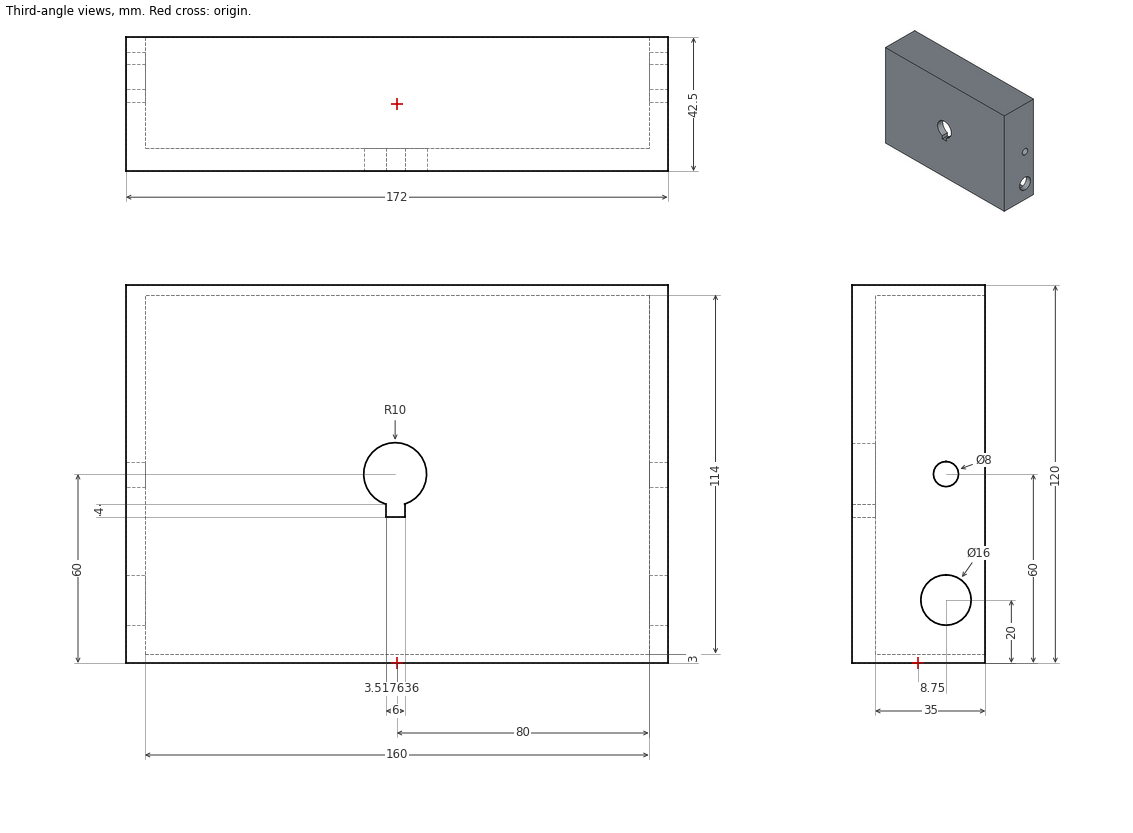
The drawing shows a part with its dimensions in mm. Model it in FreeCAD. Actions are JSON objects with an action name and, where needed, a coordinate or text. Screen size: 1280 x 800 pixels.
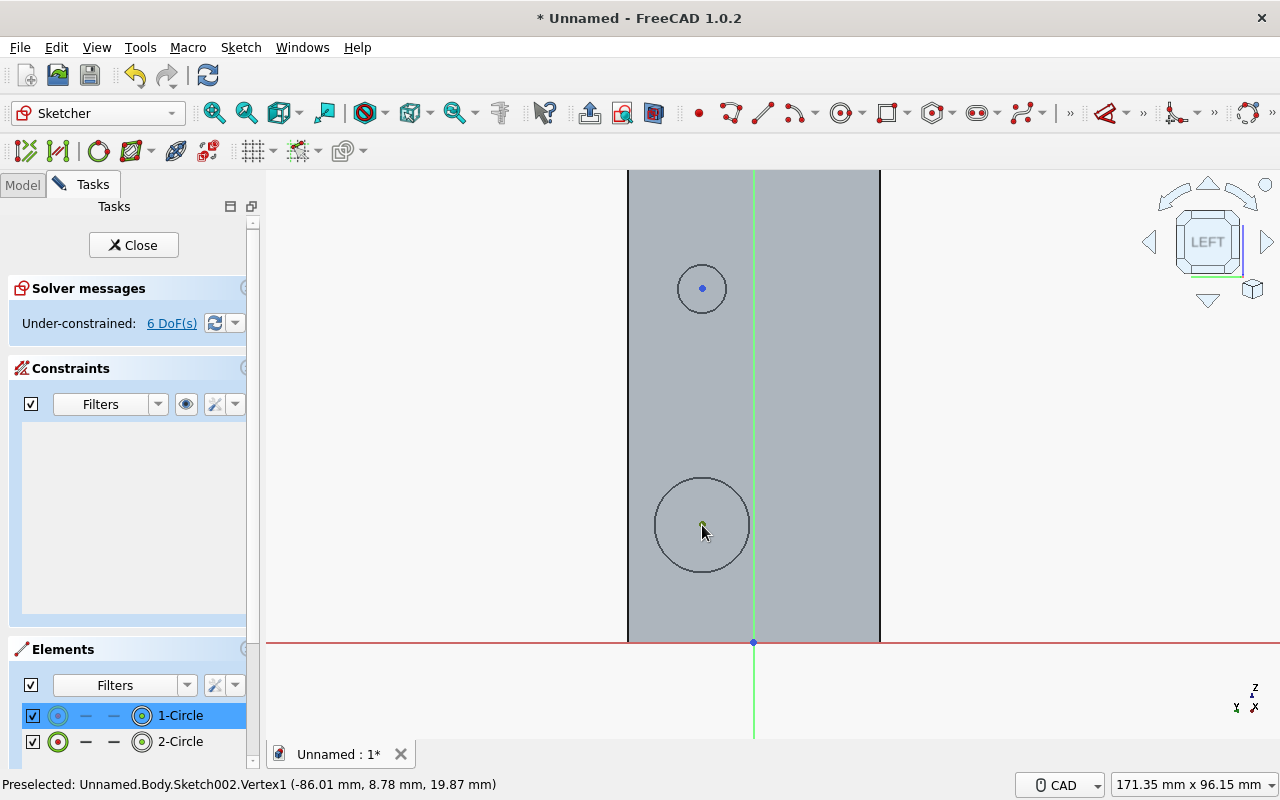
{"action": "left_click", "coordinate": [702, 289]}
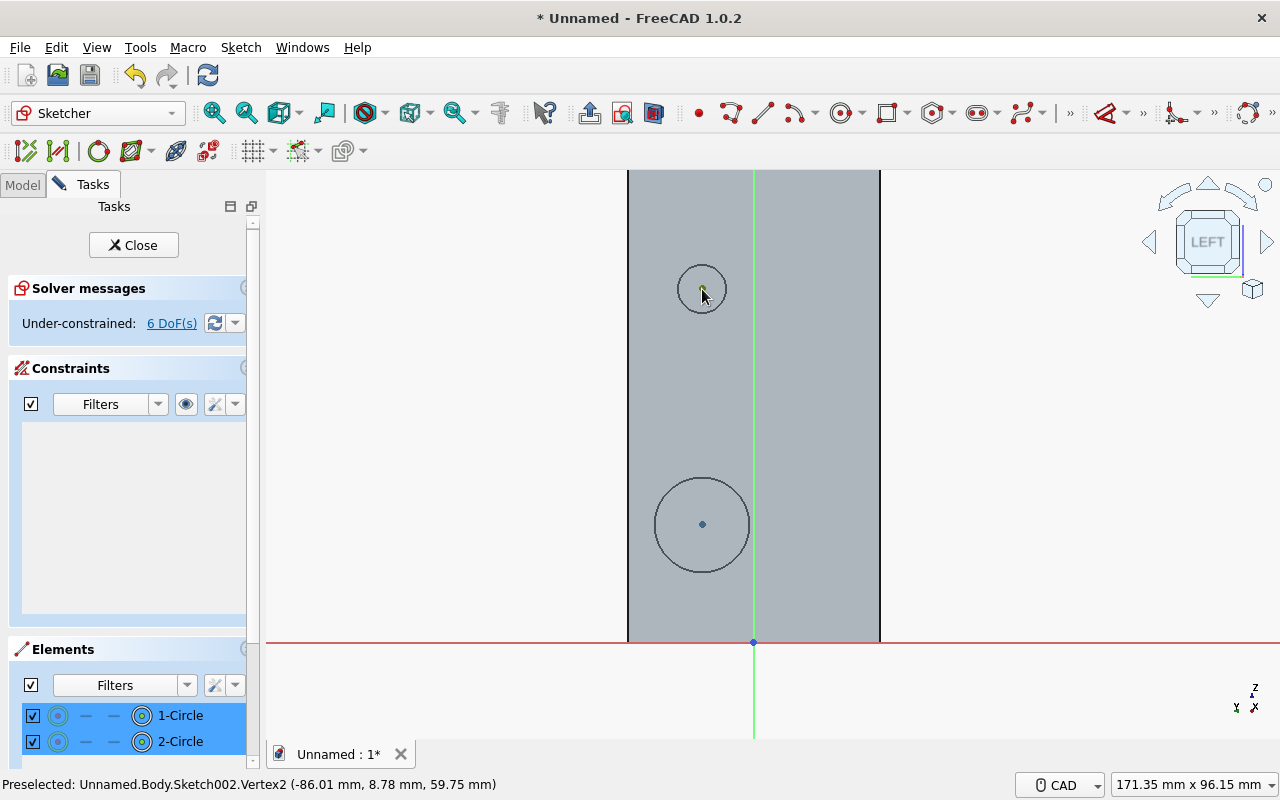
{"action": "key", "text": "v"}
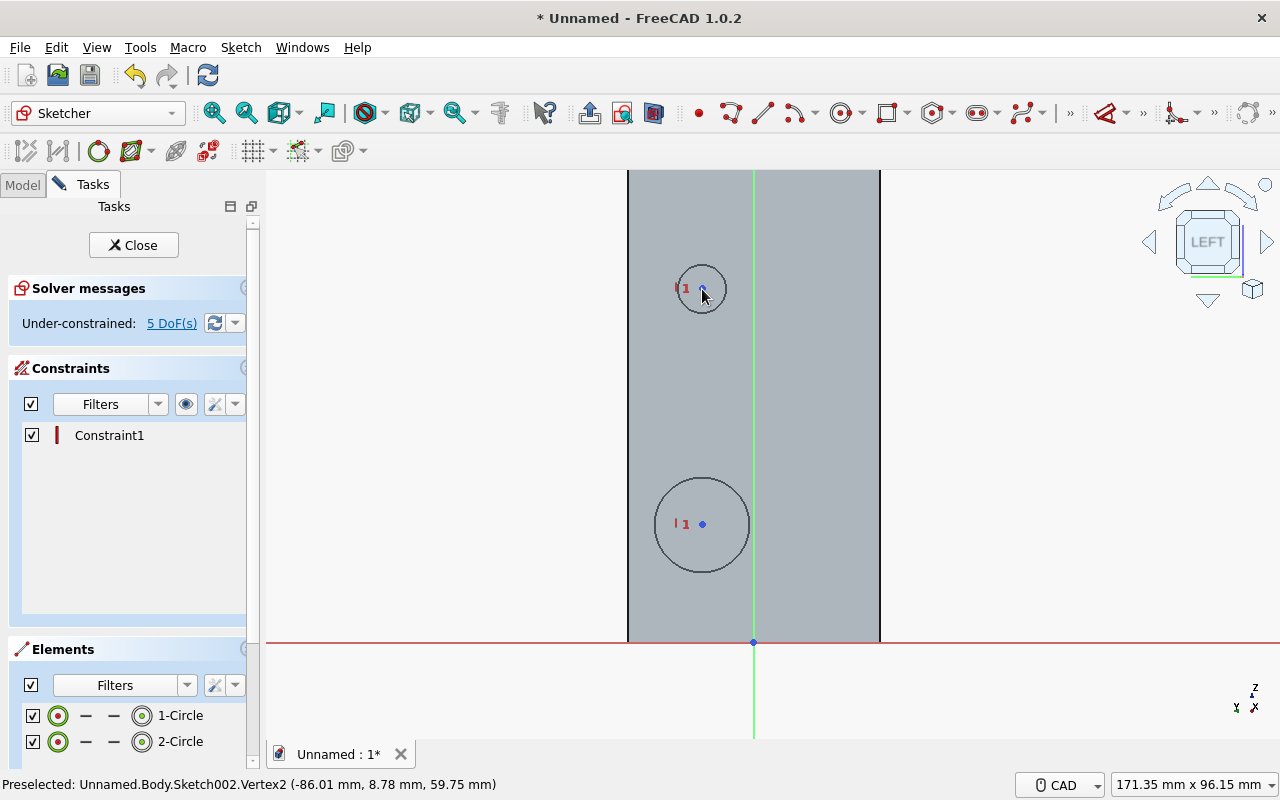
{"action": "left_click", "coordinate": [1106, 114]}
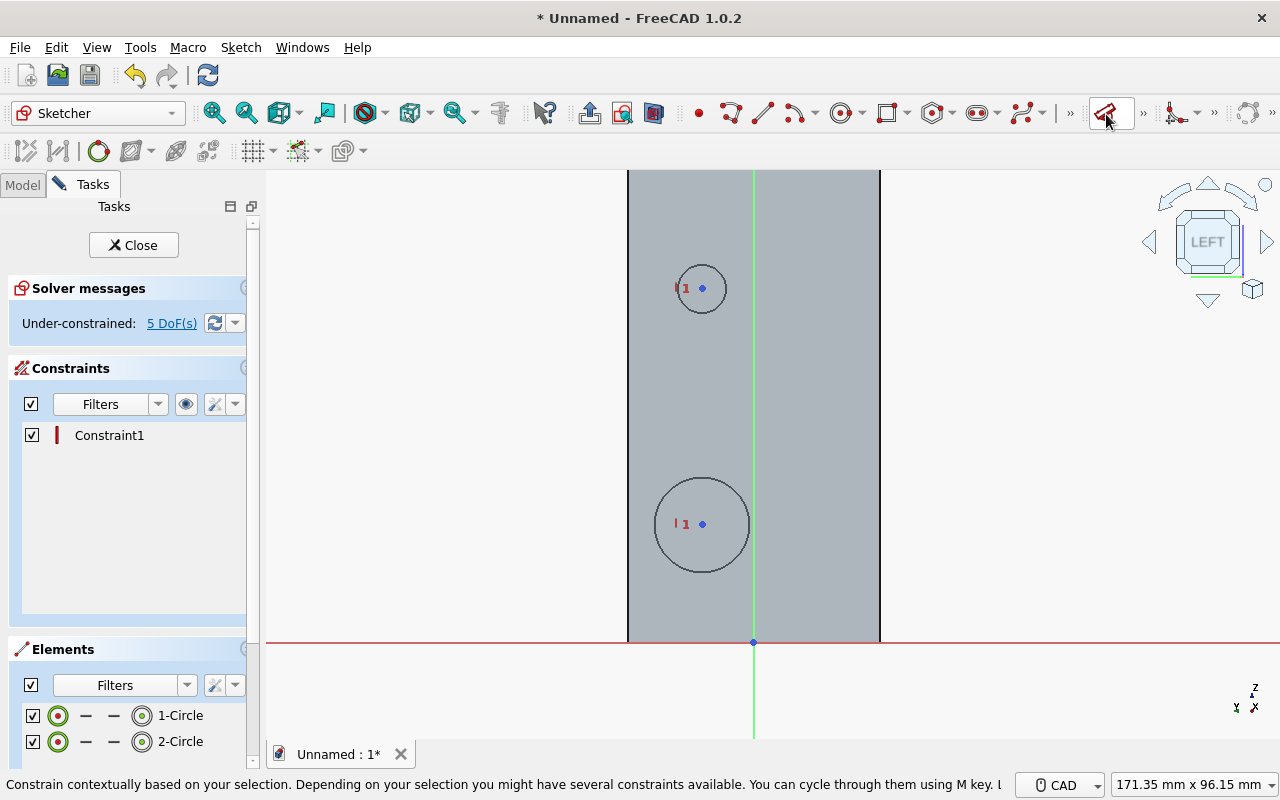
{"action": "left_click", "coordinate": [735, 491]}
{"action": "left_click", "coordinate": [778, 502]}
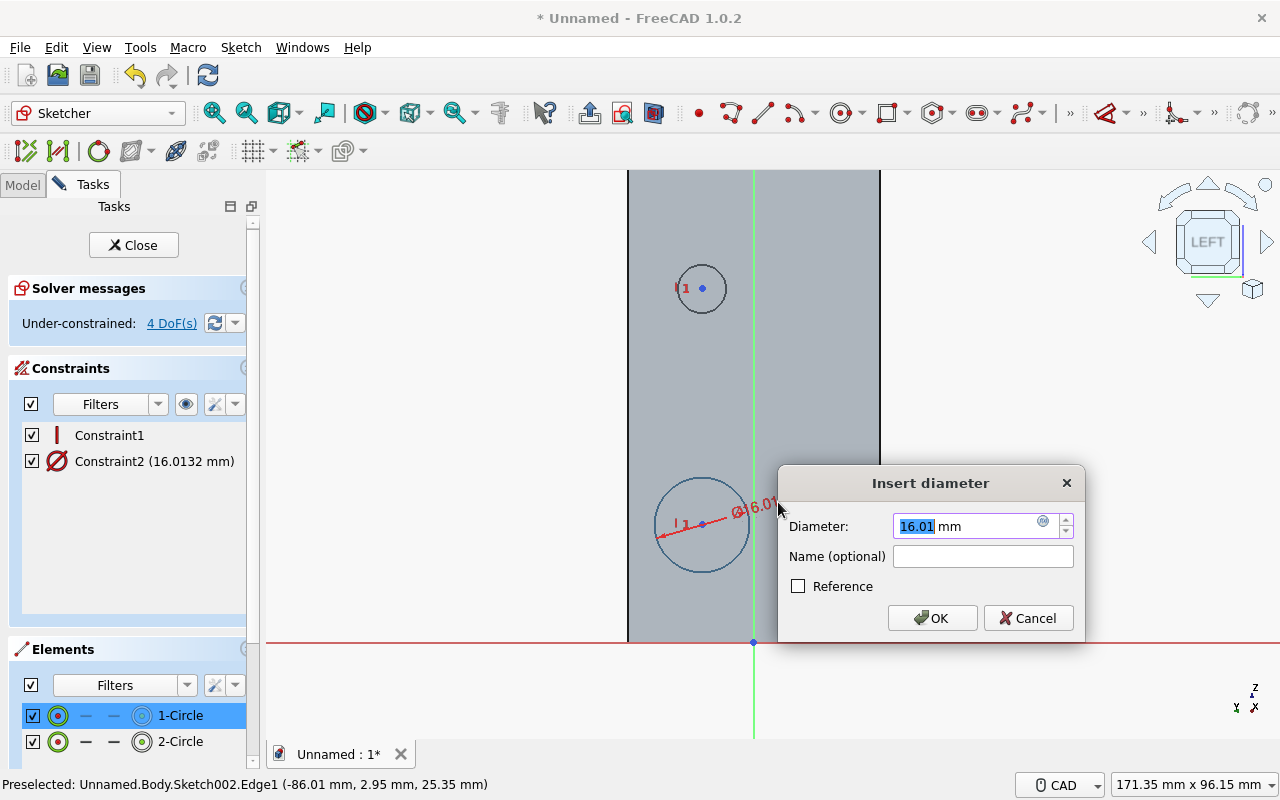
{"action": "type", "text": "16"}
{"action": "key", "text": "Return"}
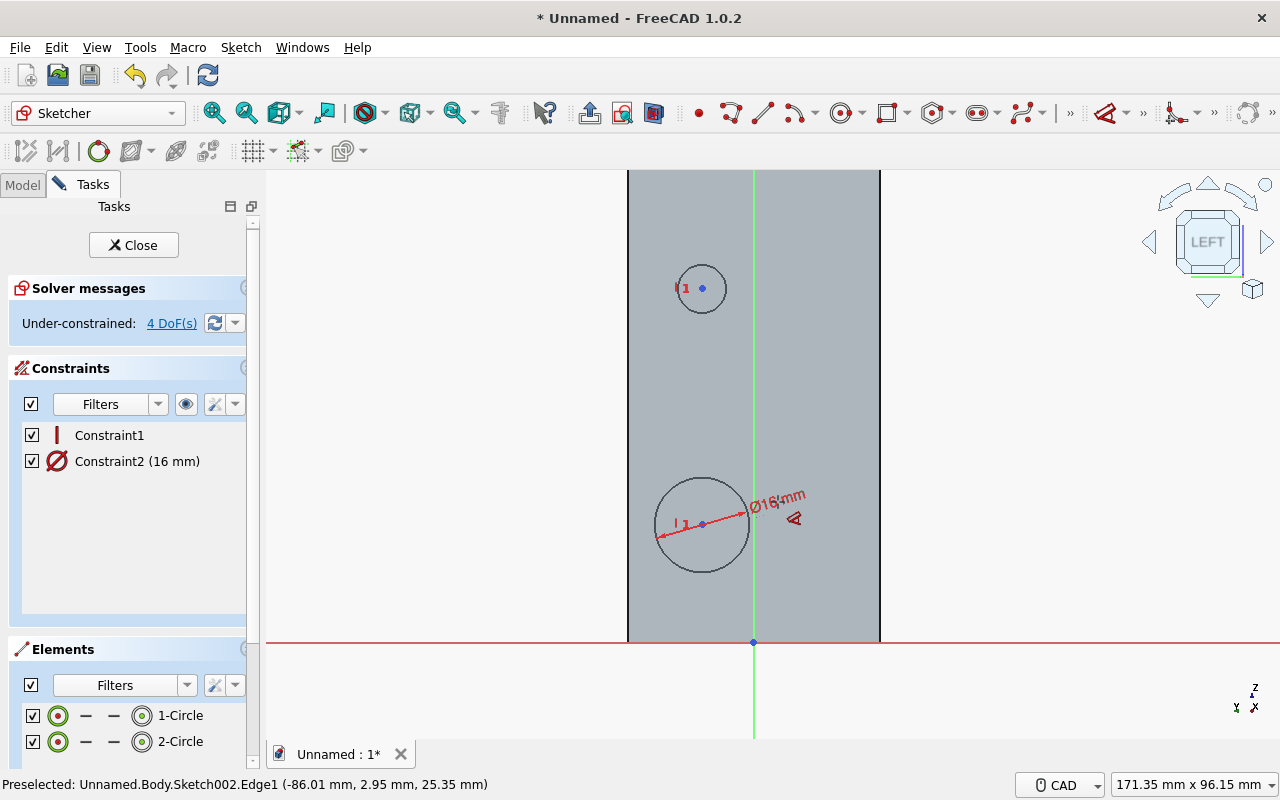
{"action": "left_click", "coordinate": [719, 272]}
{"action": "left_click", "coordinate": [718, 235]}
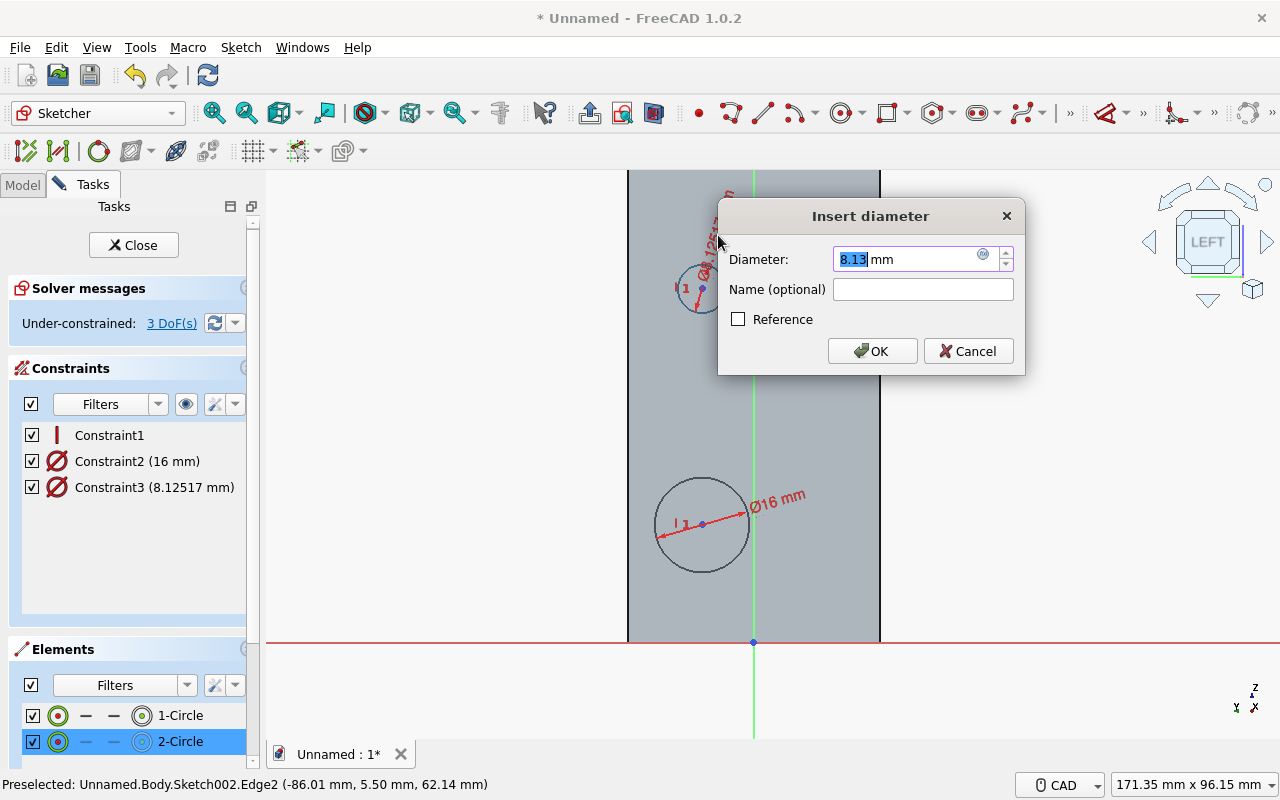
{"action": "type", "text": "8"}
{"action": "key", "text": "Return"}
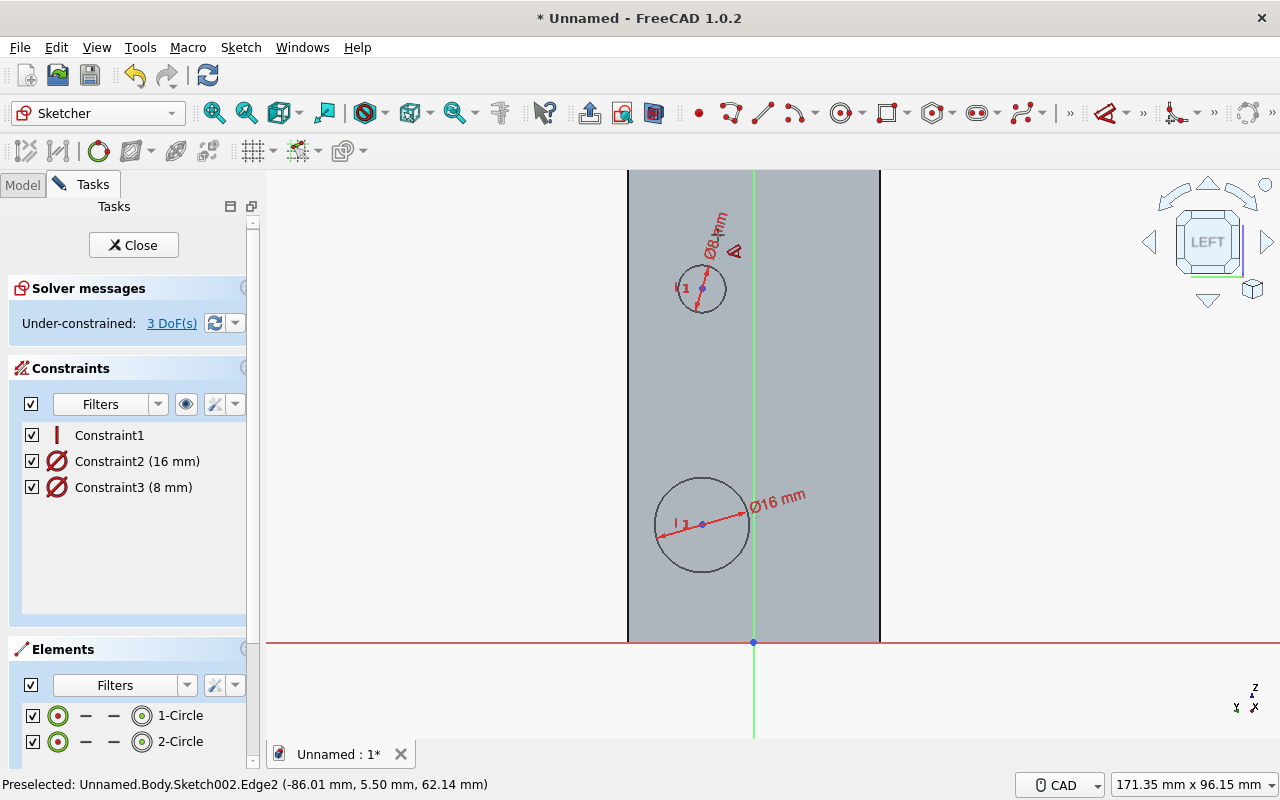
{"action": "left_click", "coordinate": [702, 525]}
{"action": "left_click", "coordinate": [788, 584]}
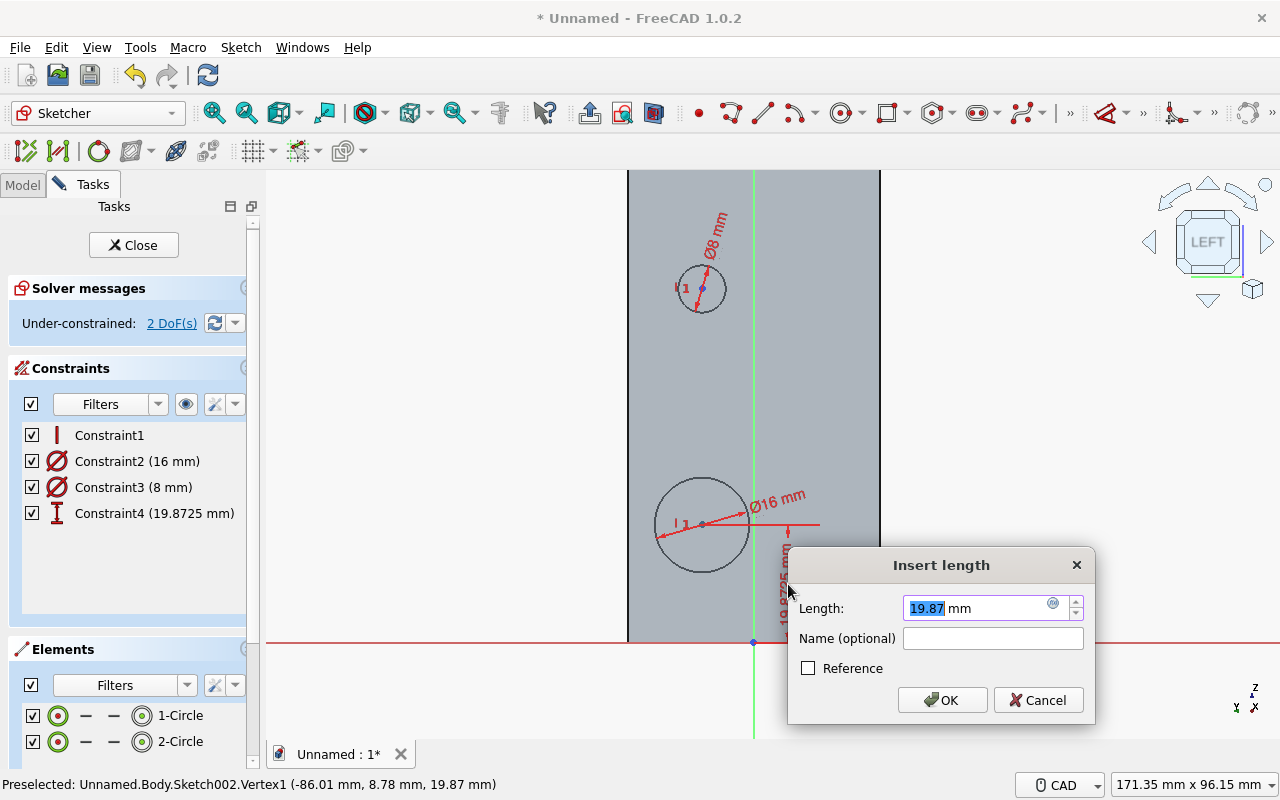
{"action": "type", "text": "20"}
{"action": "key", "text": "Return"}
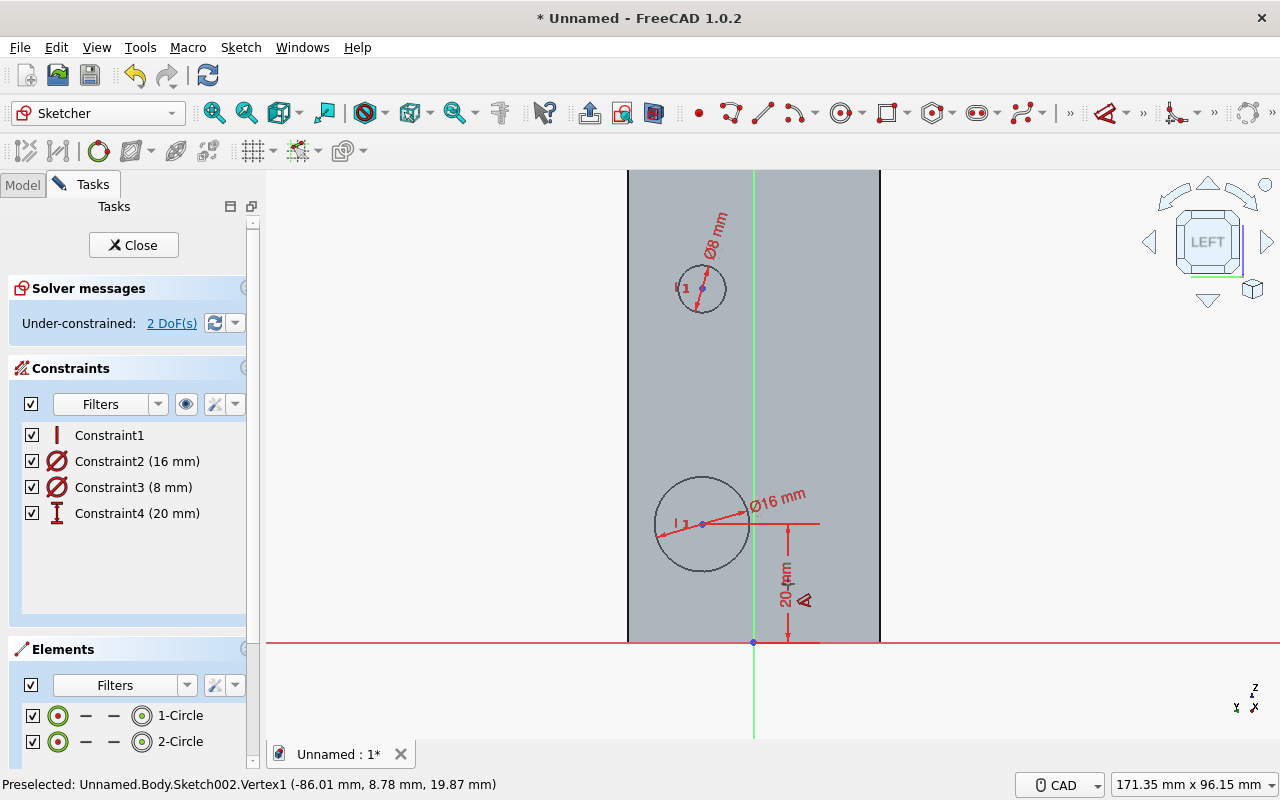
{"action": "left_click", "coordinate": [702, 289]}
{"action": "left_click", "coordinate": [788, 466]}